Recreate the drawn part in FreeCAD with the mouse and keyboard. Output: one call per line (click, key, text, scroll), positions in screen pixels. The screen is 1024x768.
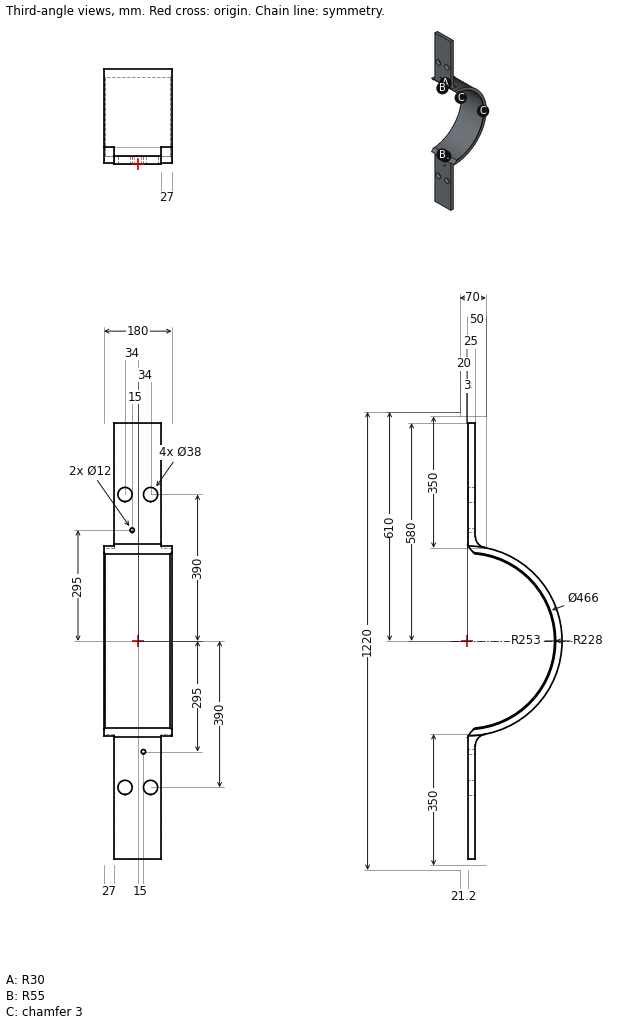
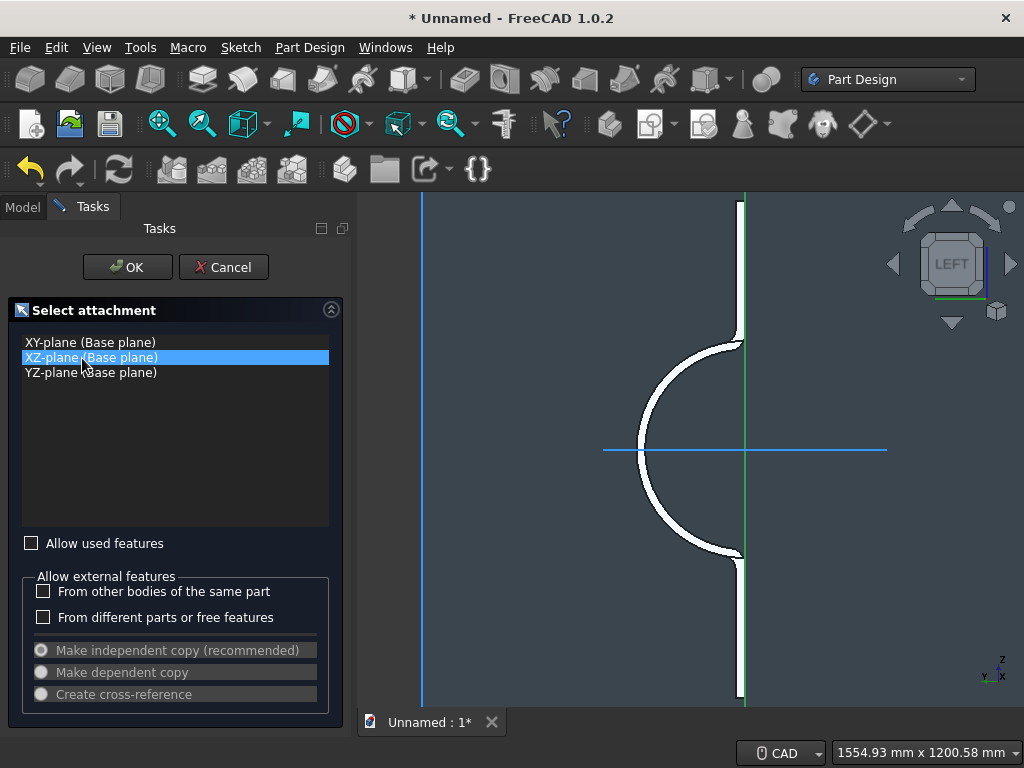
click(128, 267)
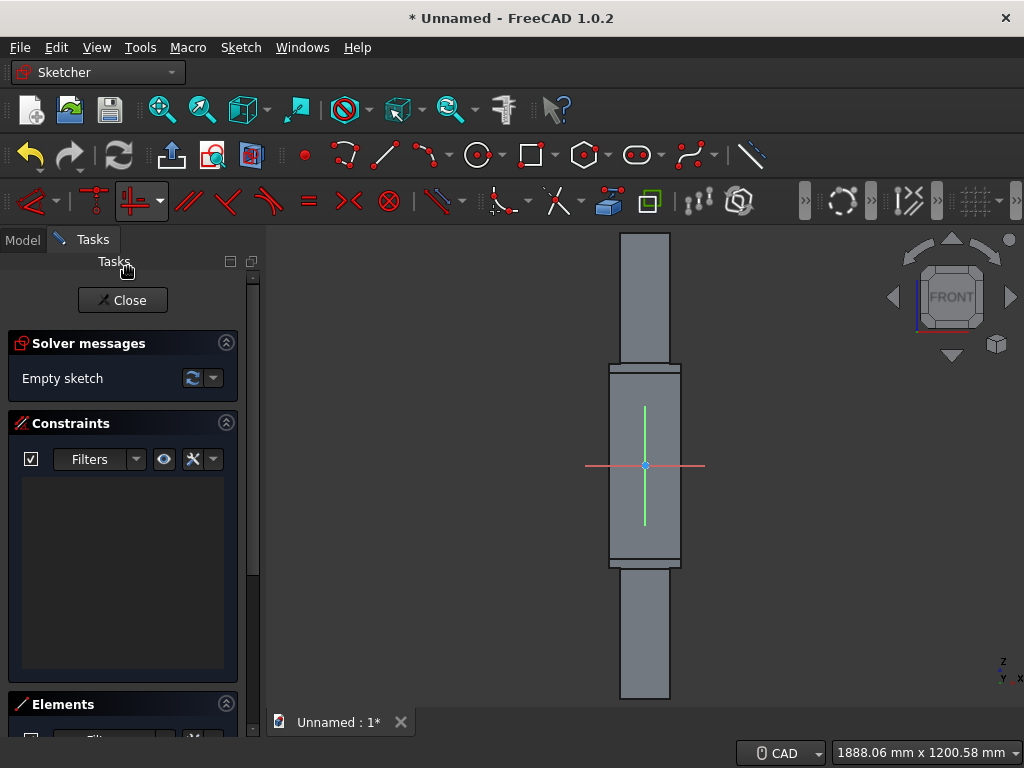
click(478, 156)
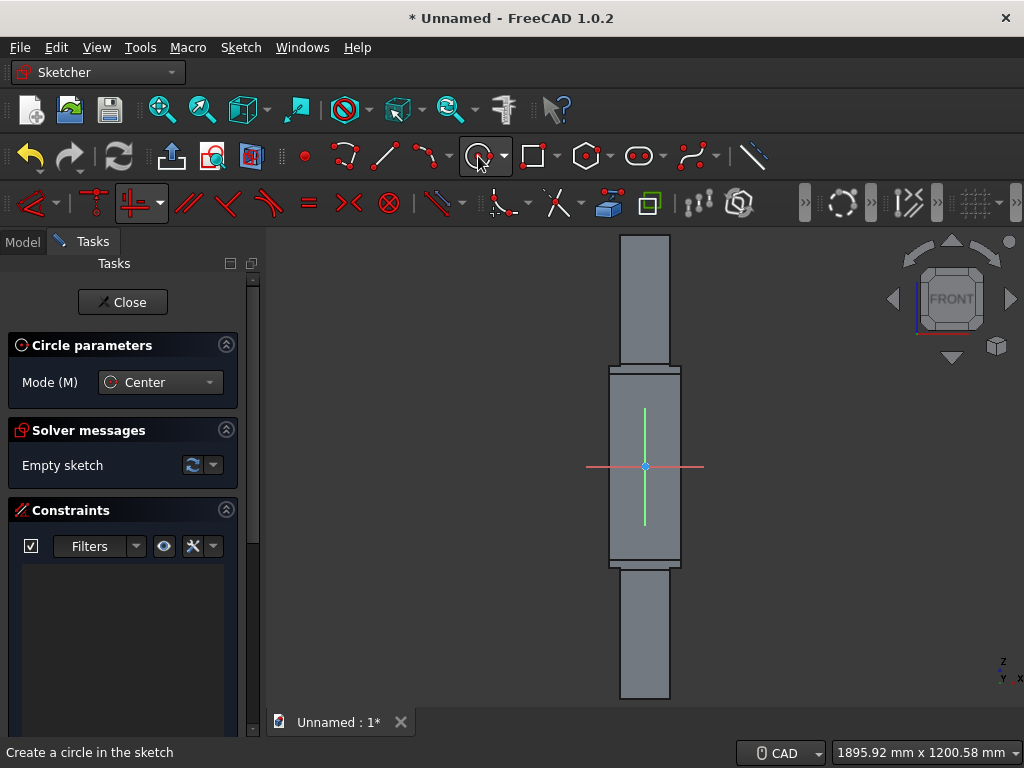
scroll(659, 311, up, 6)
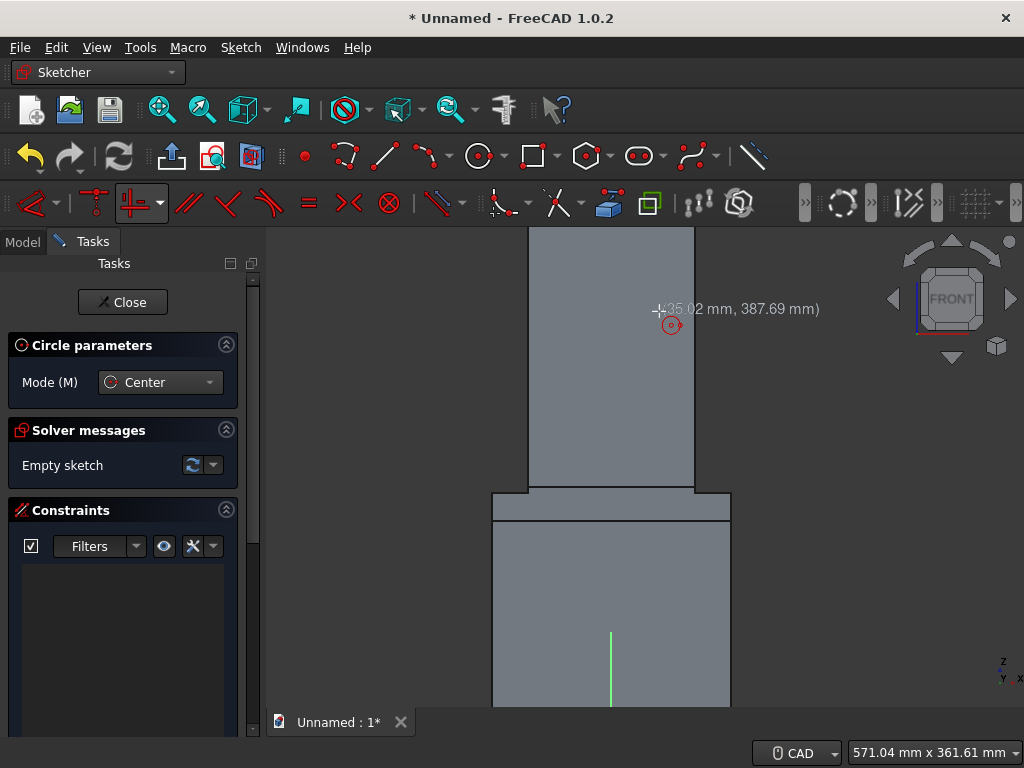
click(656, 311)
click(674, 293)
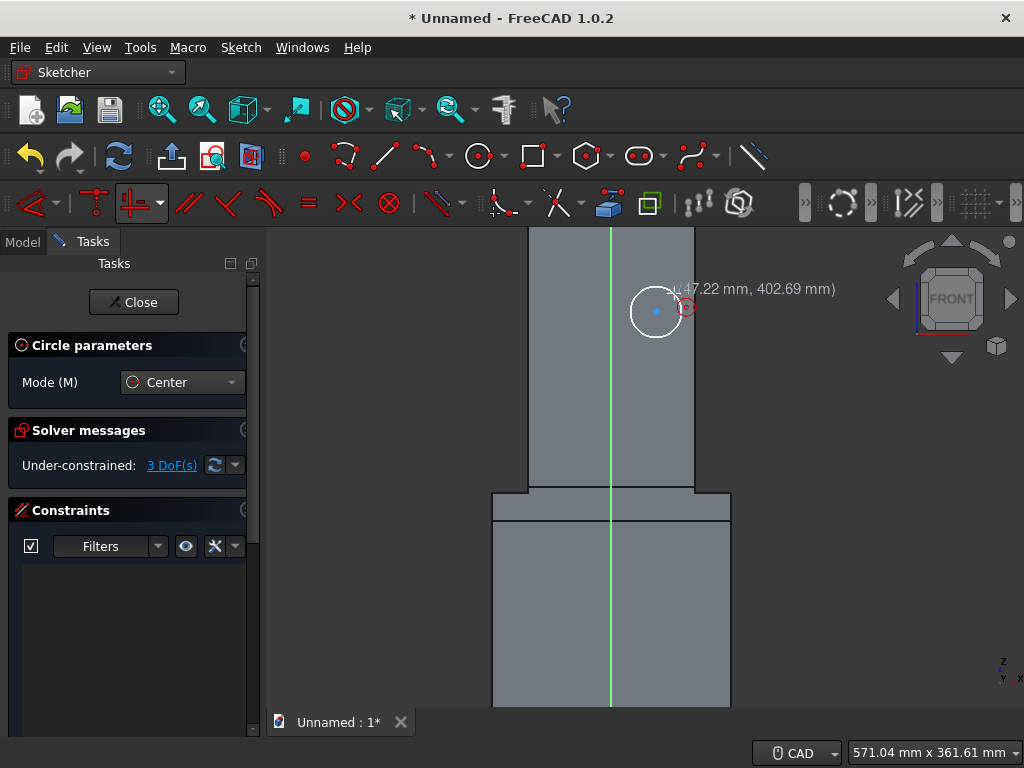
scroll(561, 311, down, 6)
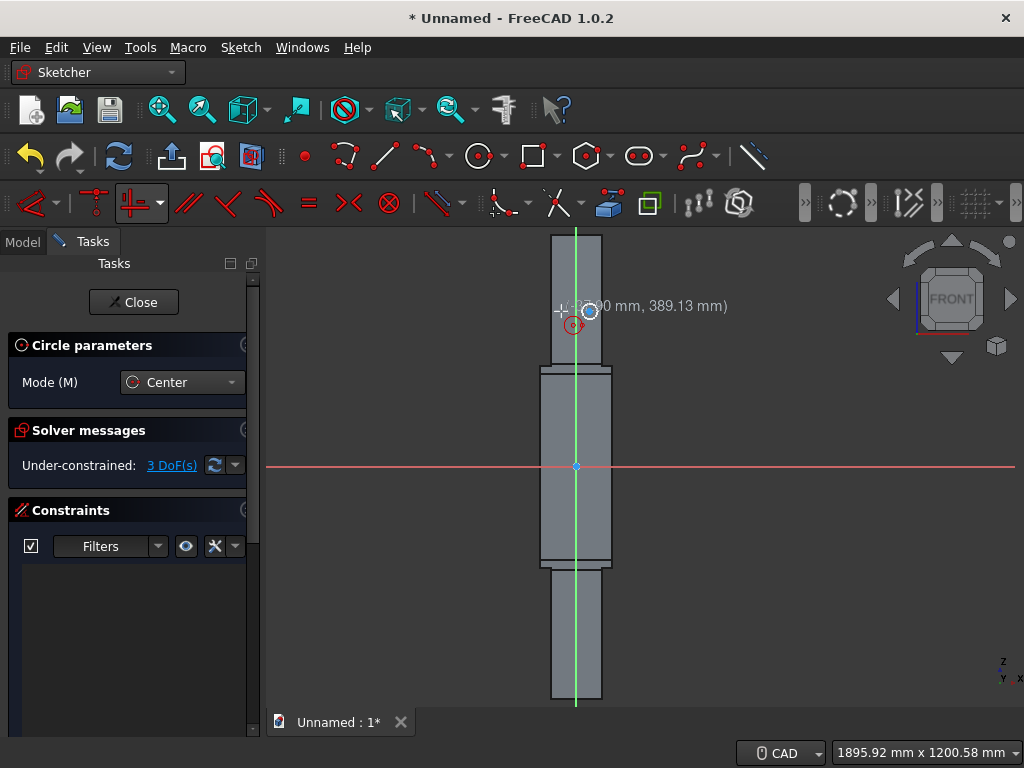
scroll(590, 623, up, 6)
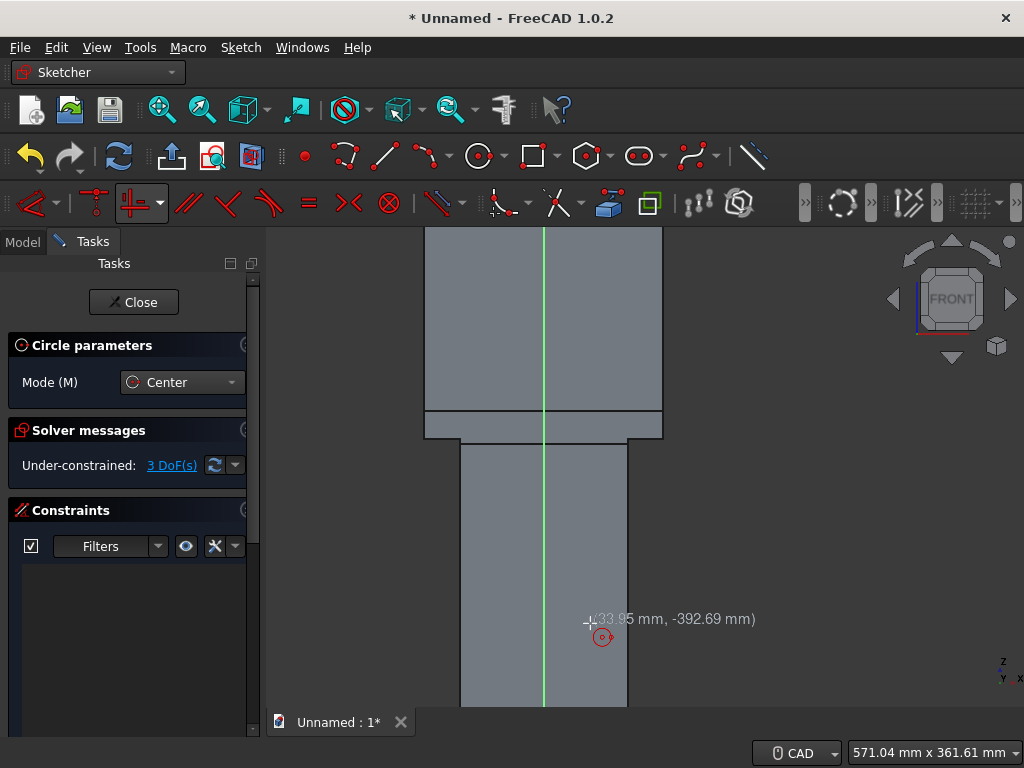
click(589, 621)
click(607, 603)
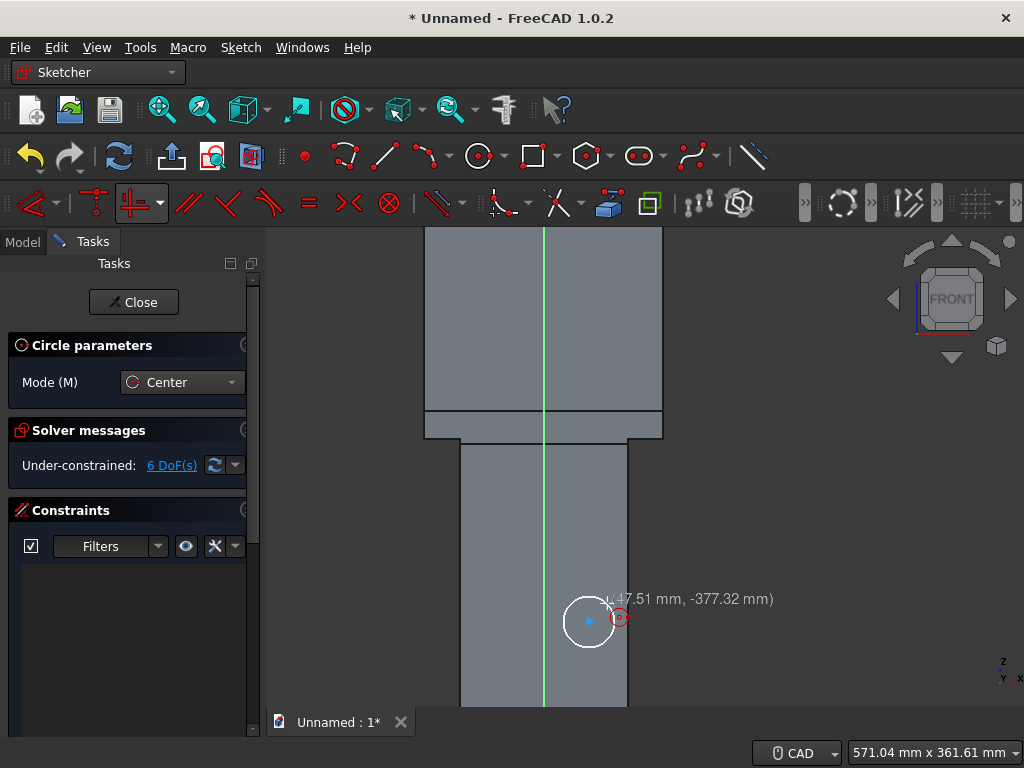
scroll(591, 624, down, 6)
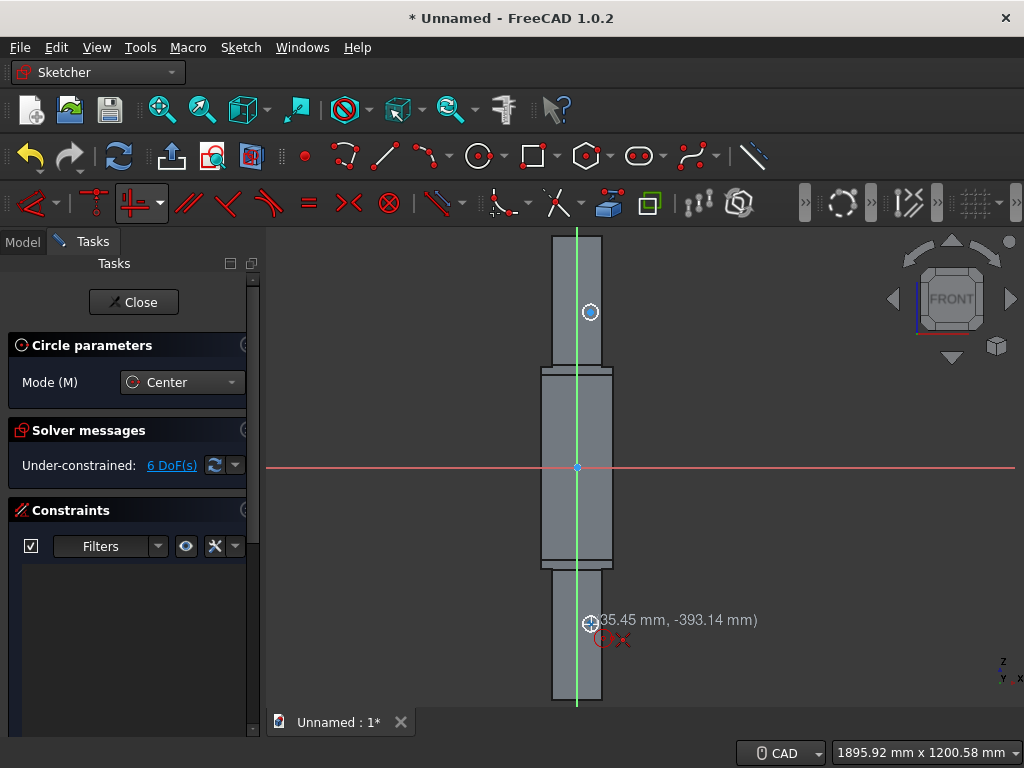
scroll(564, 312, up, 6)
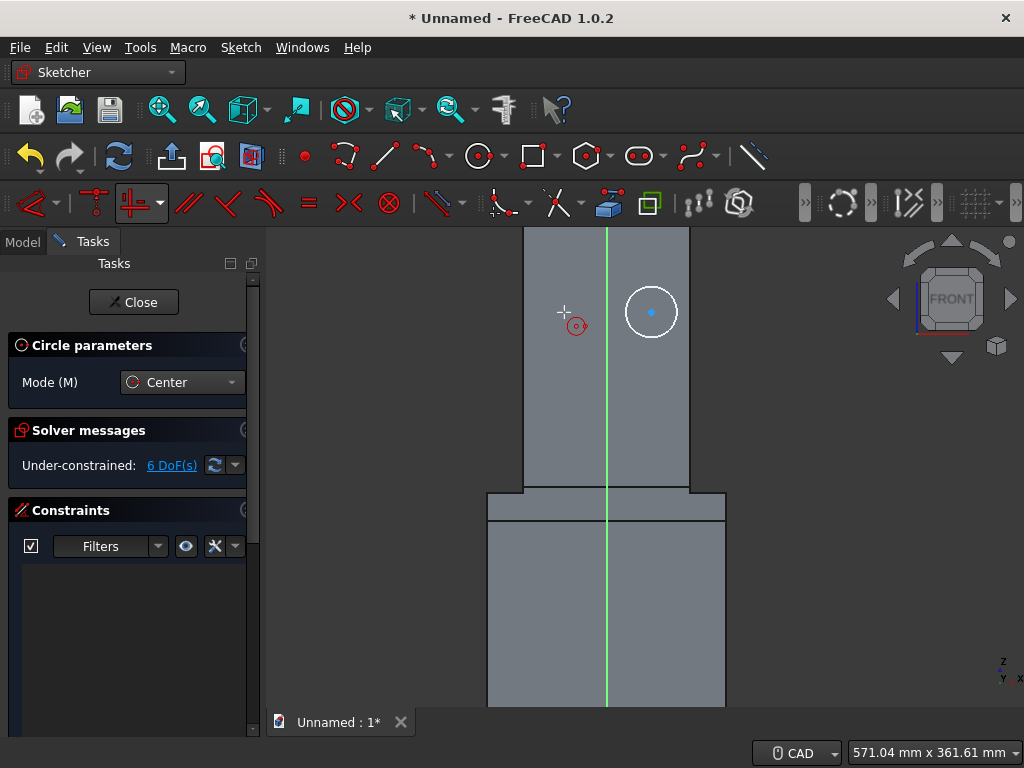
click(562, 311)
click(579, 293)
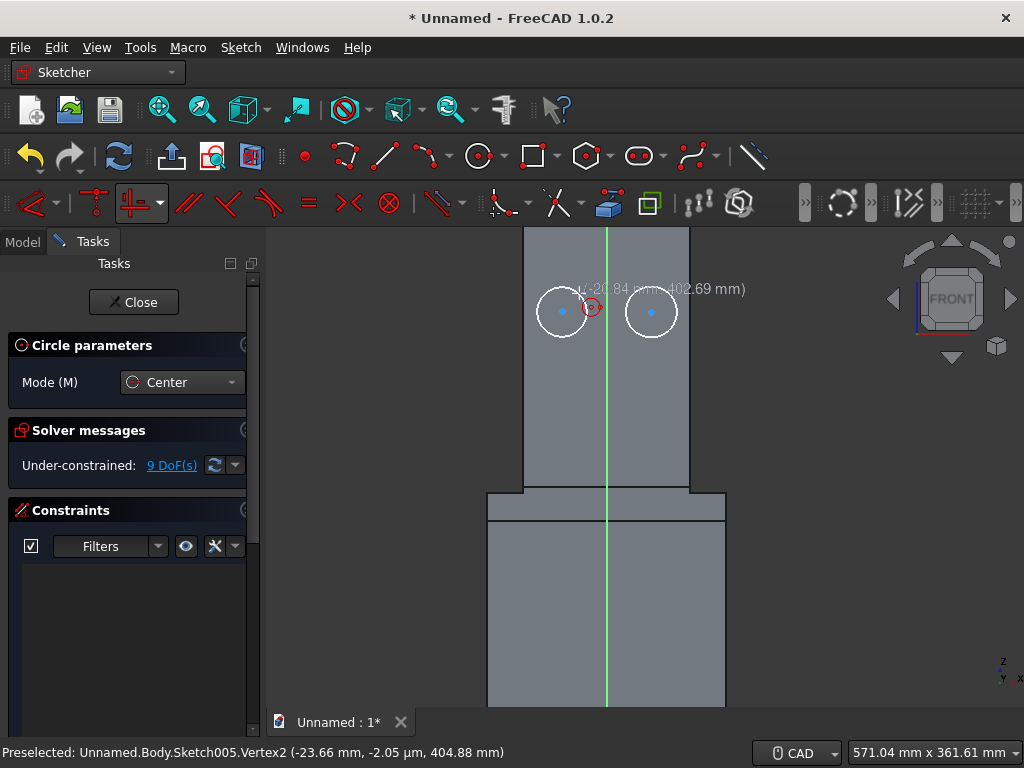
scroll(563, 311, down, 6)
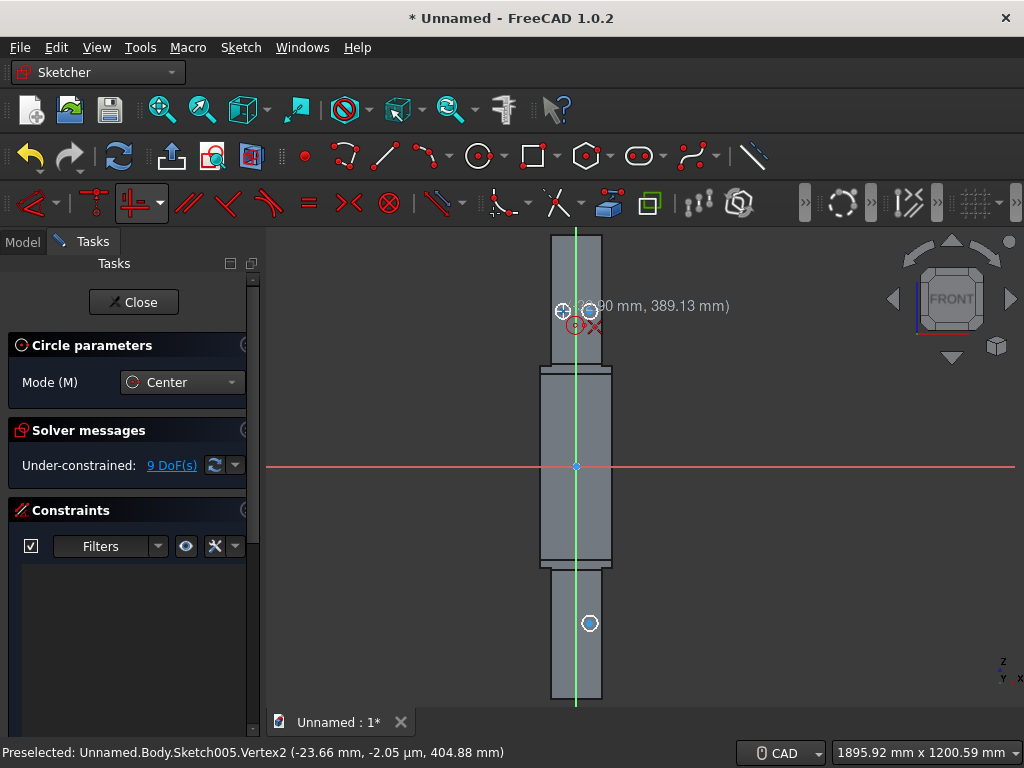
scroll(563, 623, up, 6)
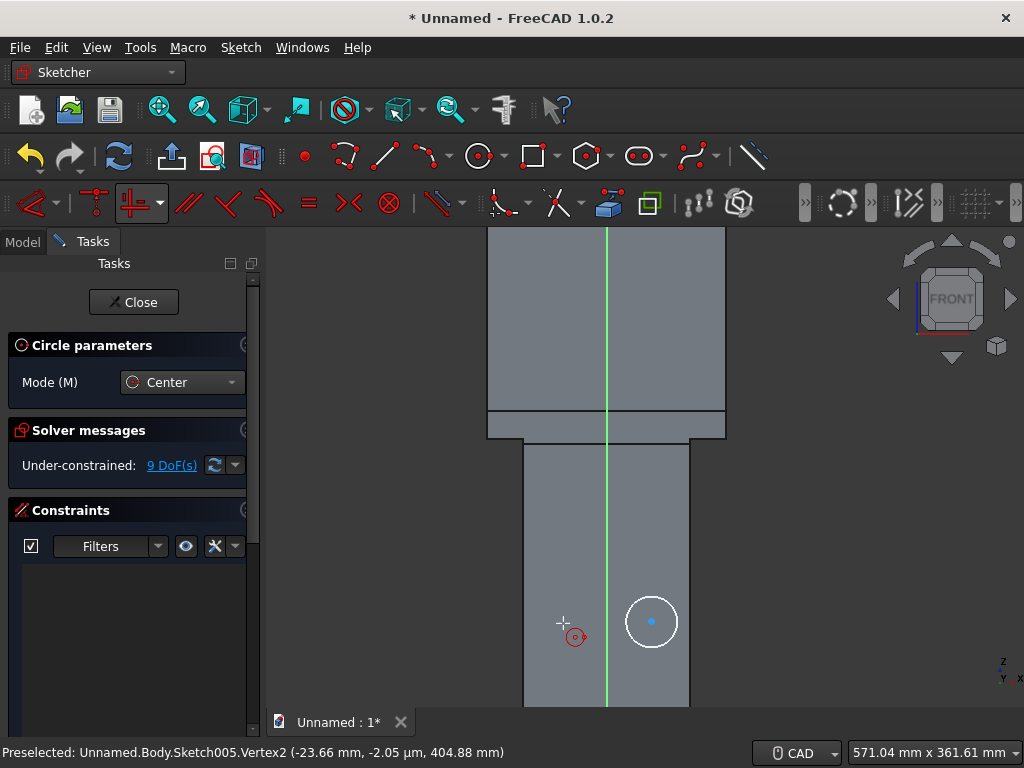
click(562, 621)
click(579, 603)